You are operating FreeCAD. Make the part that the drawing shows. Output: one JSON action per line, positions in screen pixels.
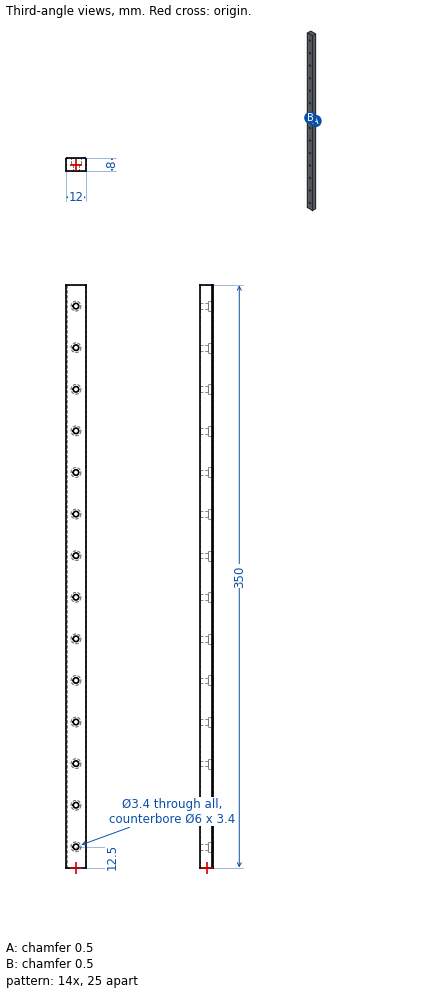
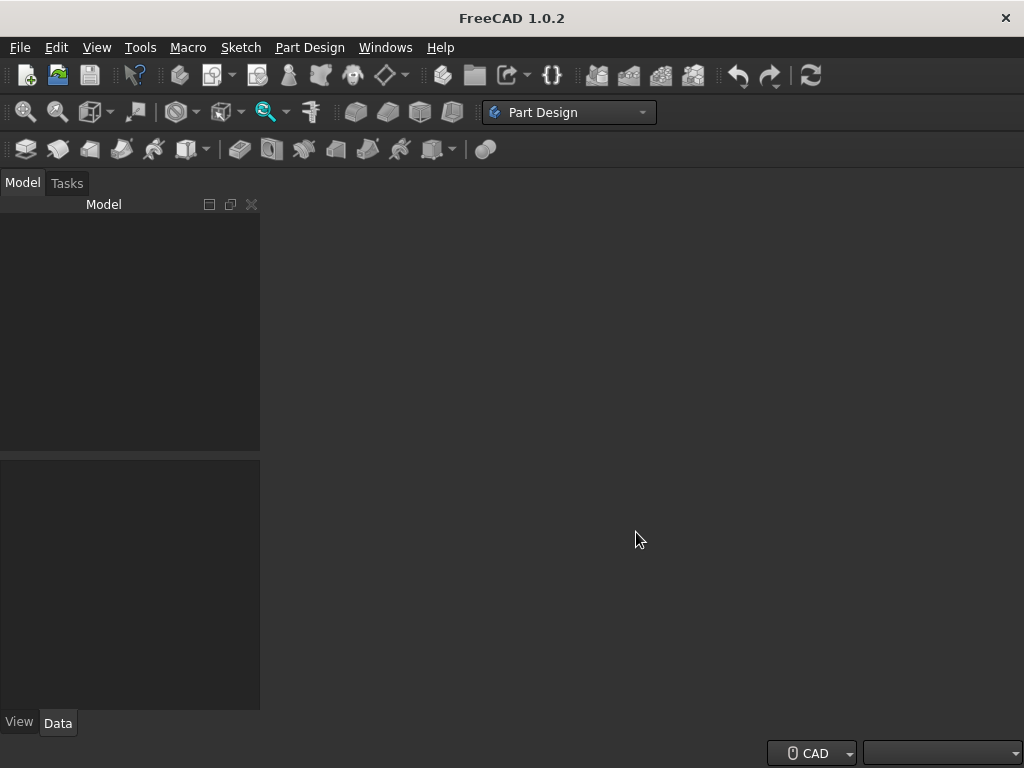
{"action": "left_click", "coordinate": [26, 76]}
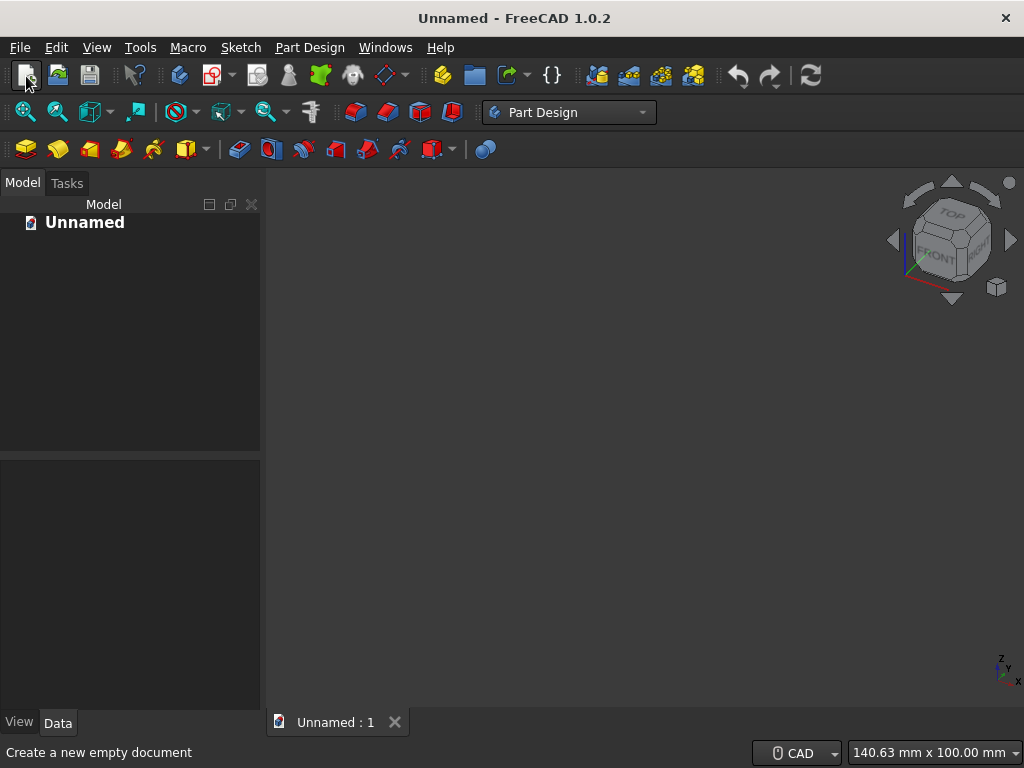
{"action": "left_click", "coordinate": [212, 76]}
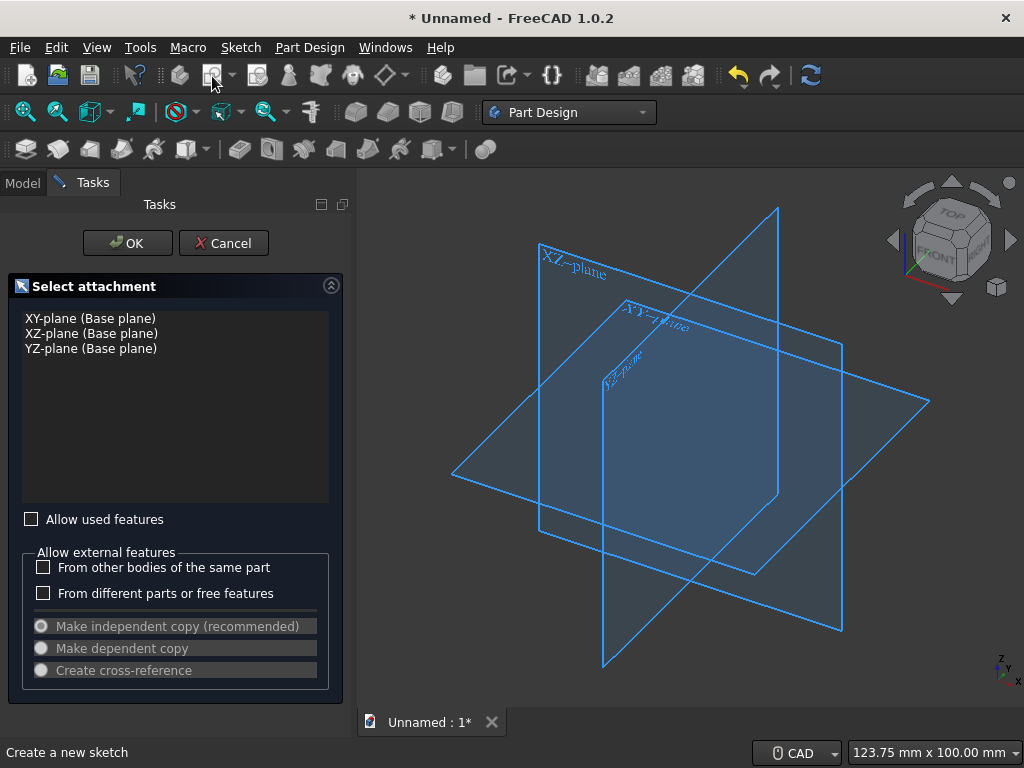
{"action": "left_click", "coordinate": [82, 318]}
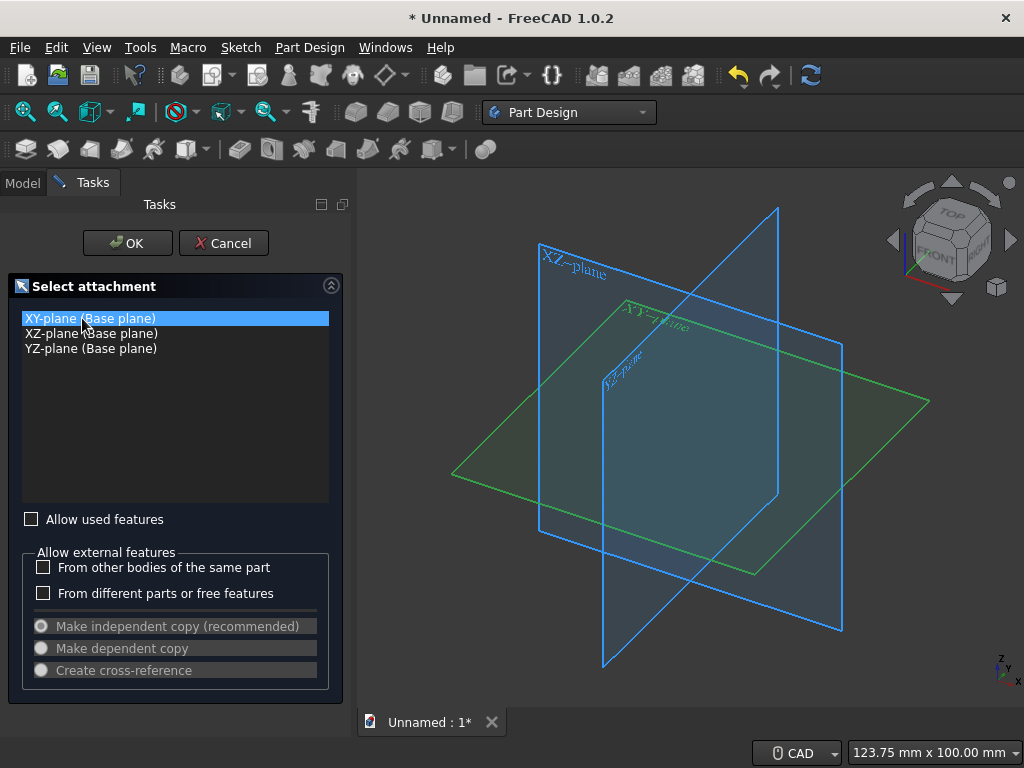
{"action": "left_click", "coordinate": [128, 243]}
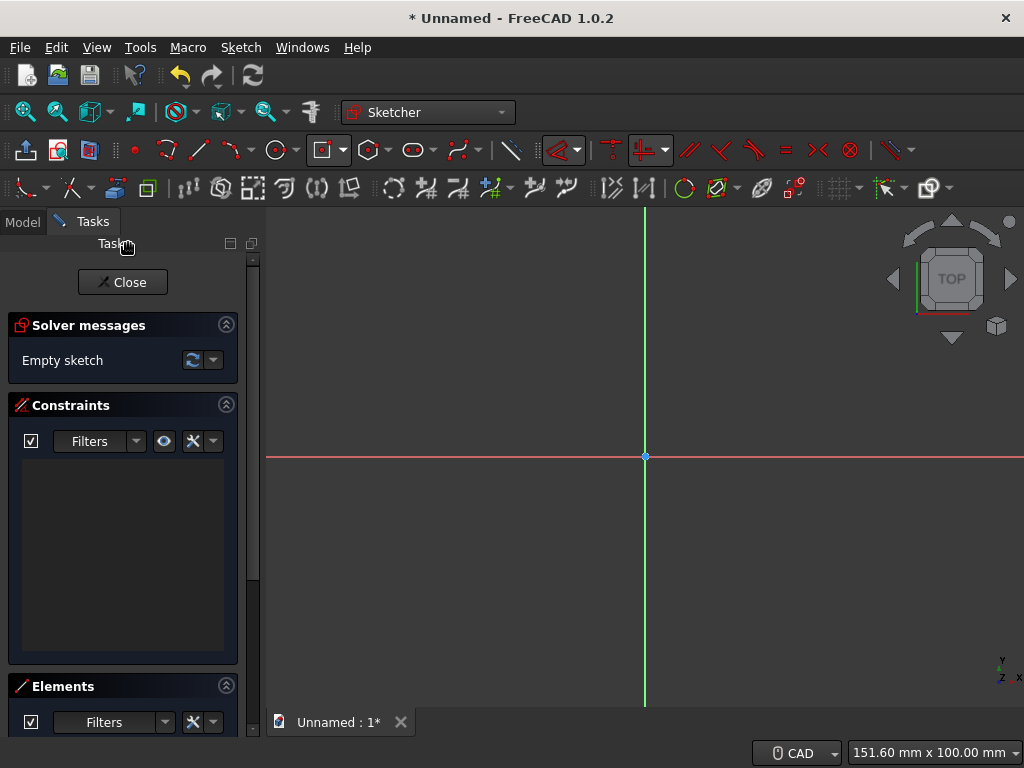
{"action": "scroll", "coordinate": [659, 457], "scroll_direction": "up", "scroll_amount": 9}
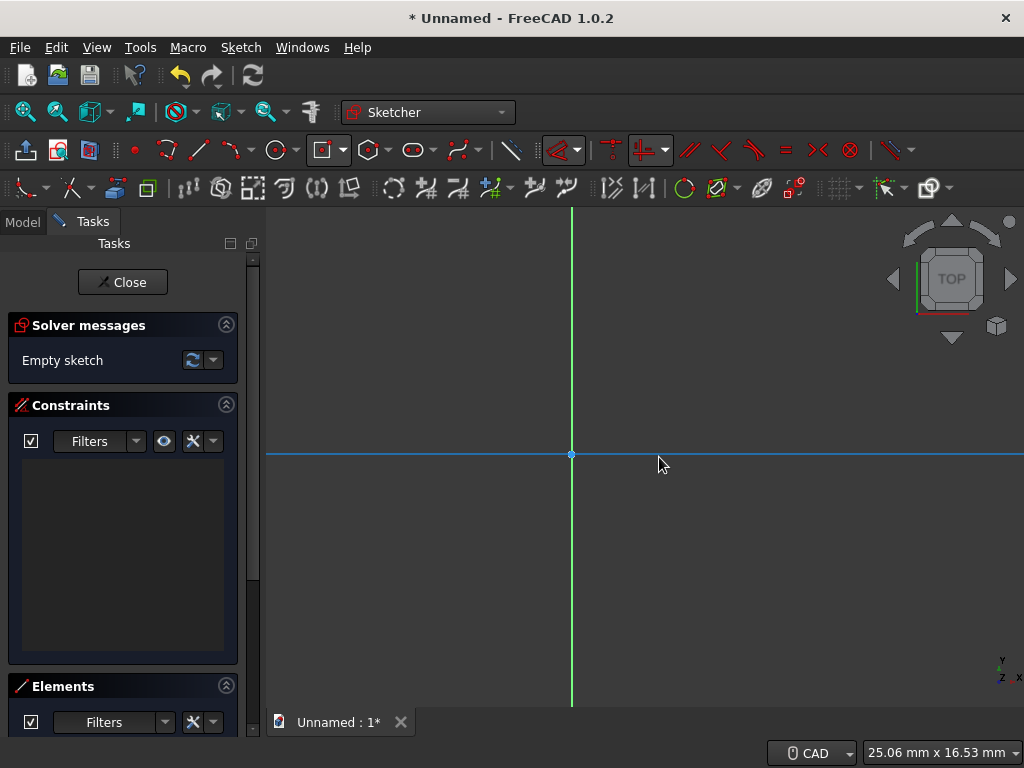
{"action": "left_click", "coordinate": [322, 150]}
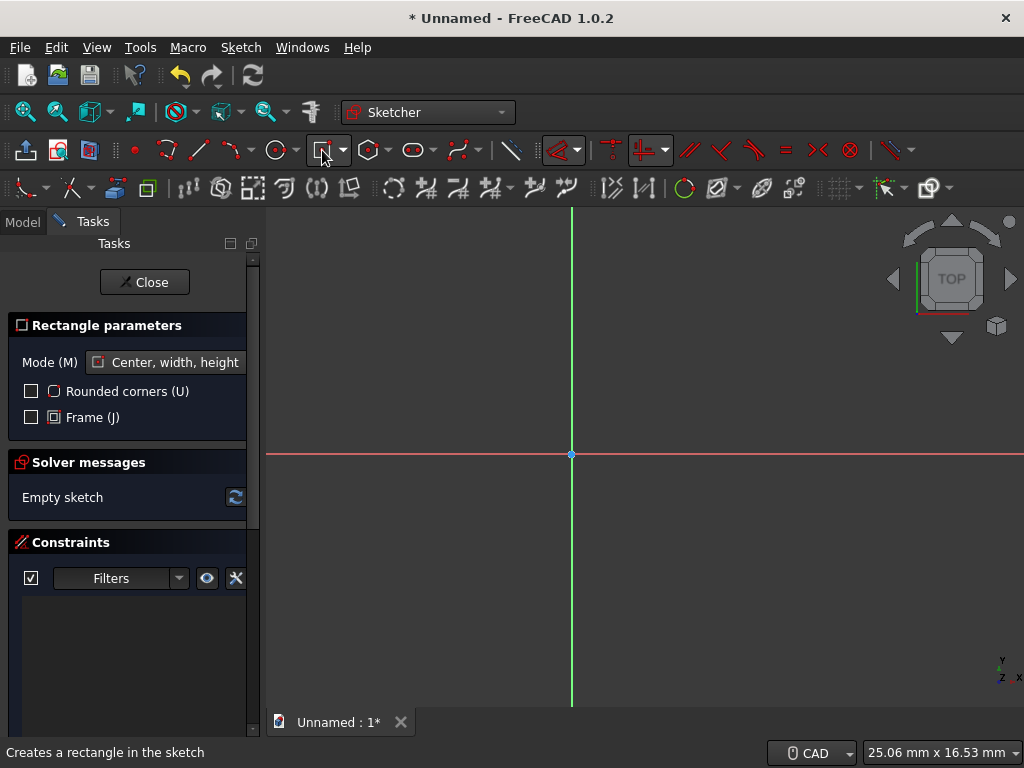
{"action": "left_click", "coordinate": [572, 454]}
{"action": "mouse_move", "coordinate": [753, 333]}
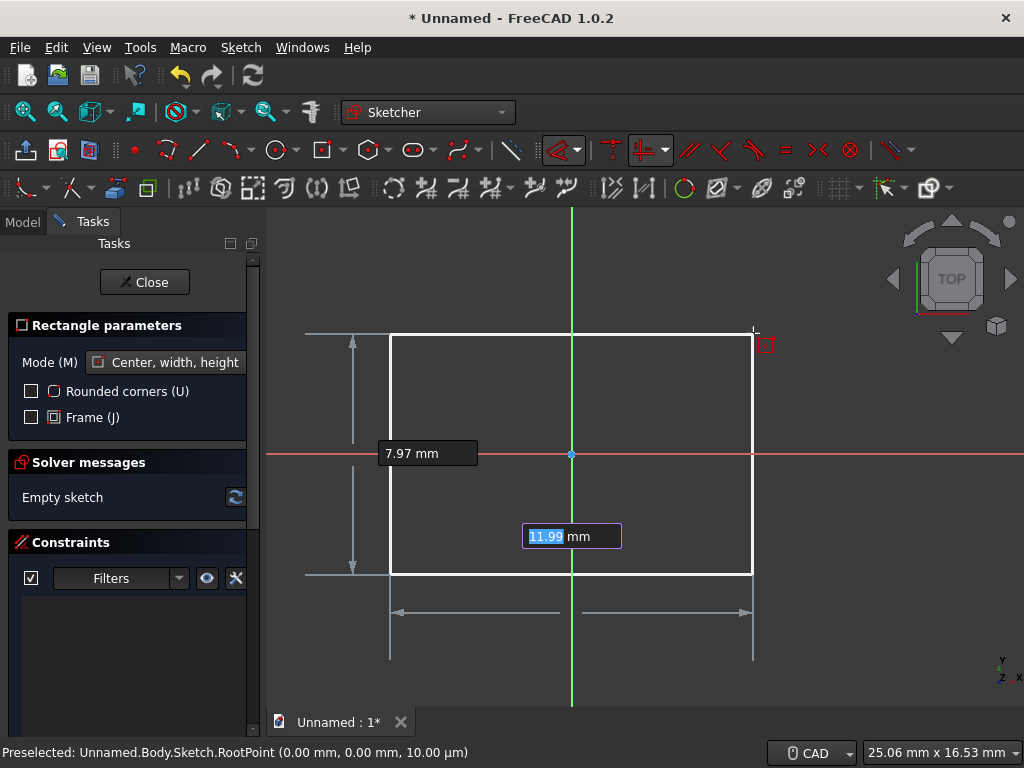
{"action": "type", "text": "12"}
{"action": "key", "text": "Tab"}
{"action": "type", "text": "8"}
{"action": "key", "text": "Return"}
{"action": "key", "text": "Escape"}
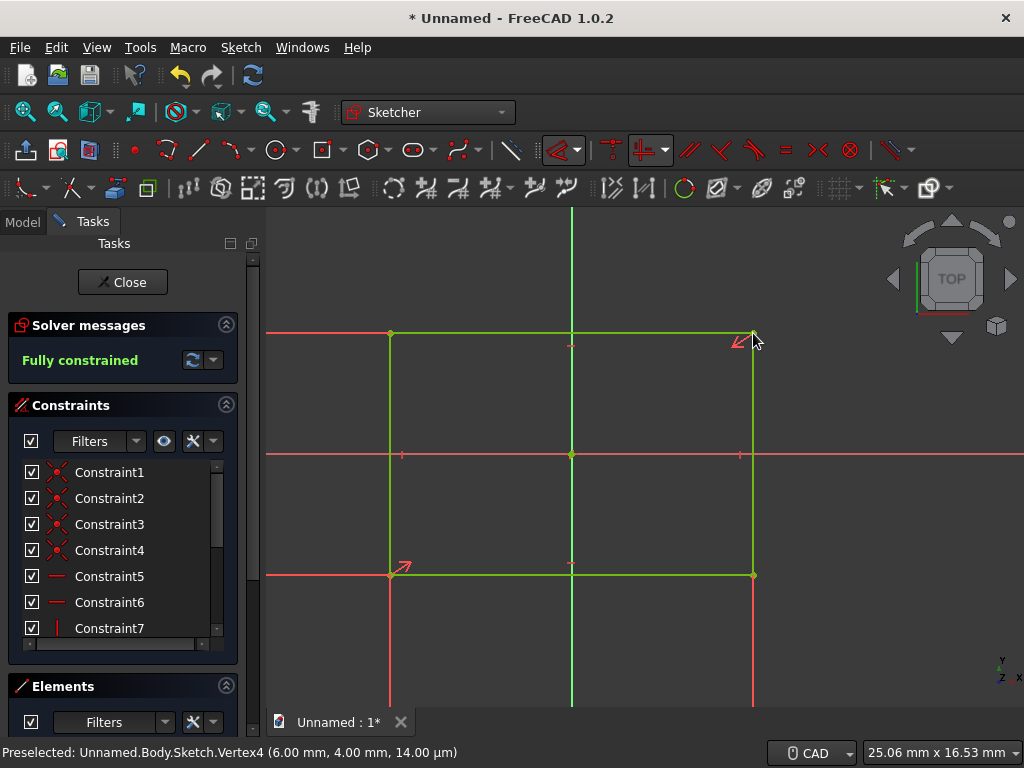
{"action": "left_click", "coordinate": [123, 282]}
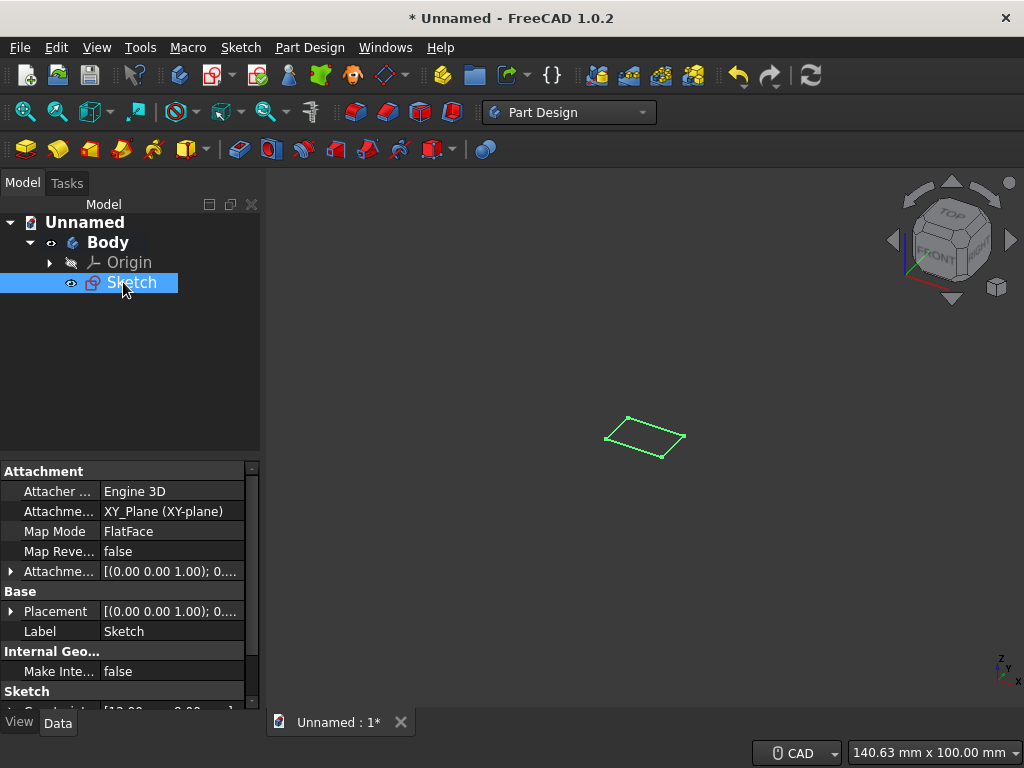
{"action": "left_click", "coordinate": [26, 150]}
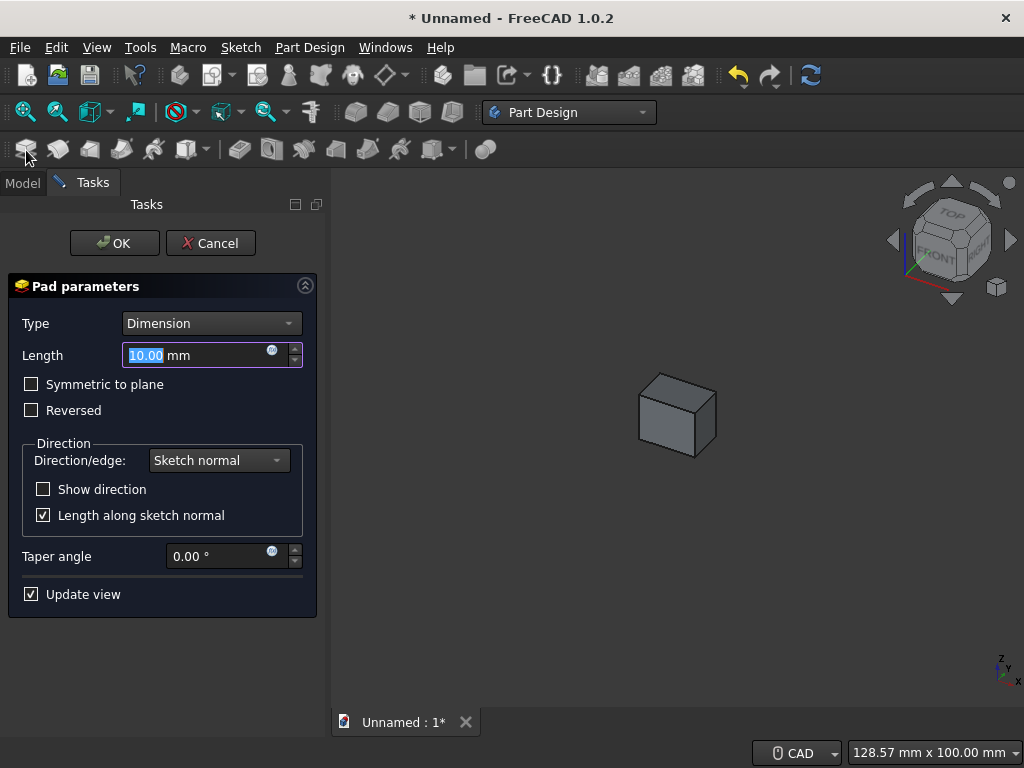
{"action": "type", "text": "350"}
{"action": "key", "text": "Tab"}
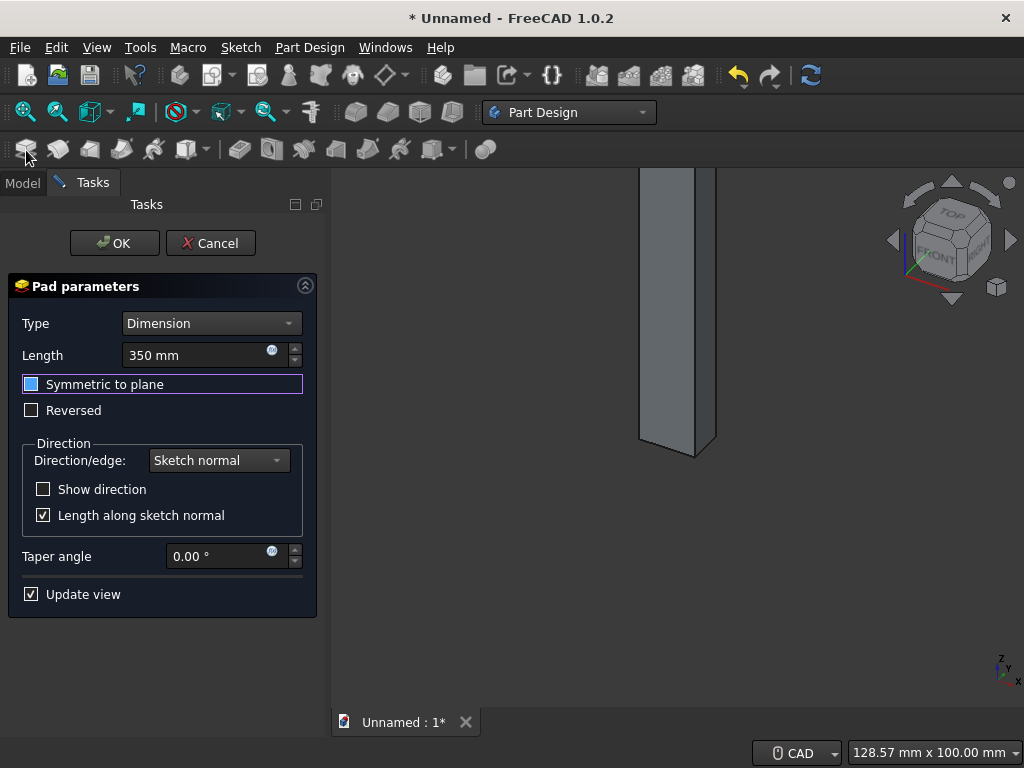
{"action": "left_click", "coordinate": [115, 243]}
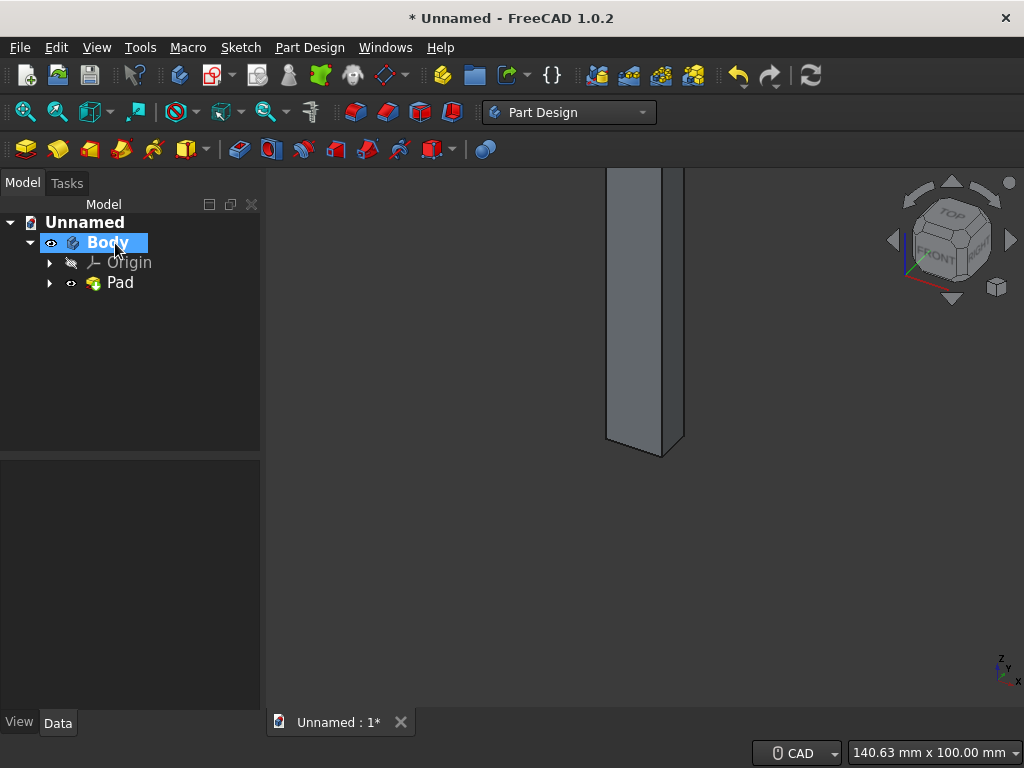
{"action": "left_click", "coordinate": [26, 112]}